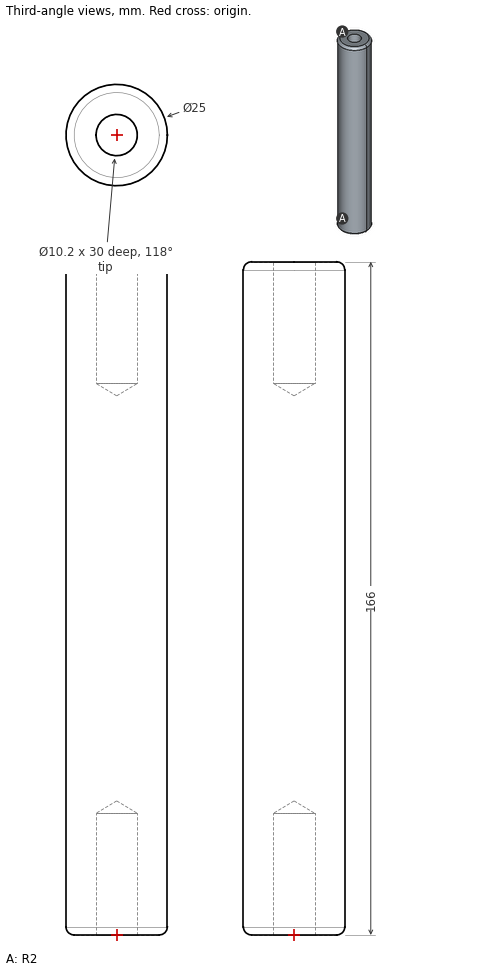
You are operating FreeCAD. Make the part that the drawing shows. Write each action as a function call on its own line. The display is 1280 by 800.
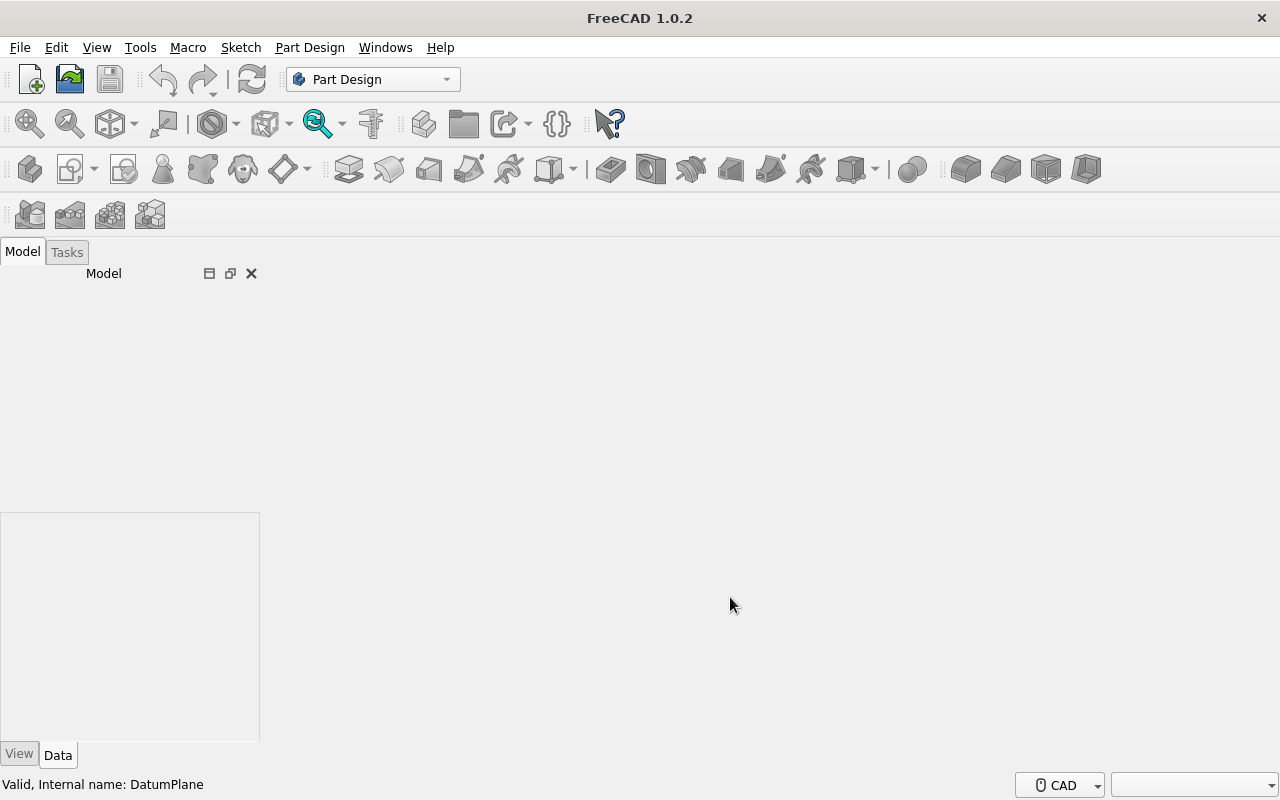
click(30, 80)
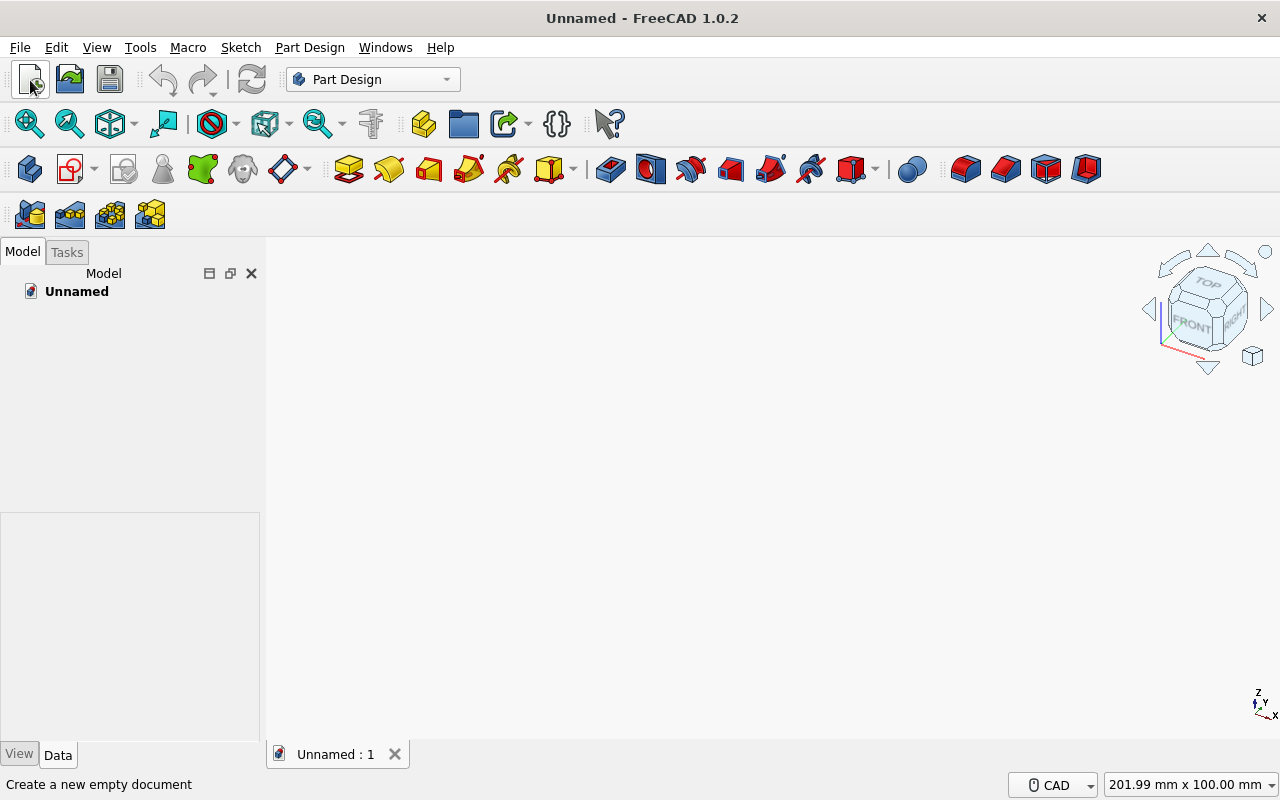
click(70, 170)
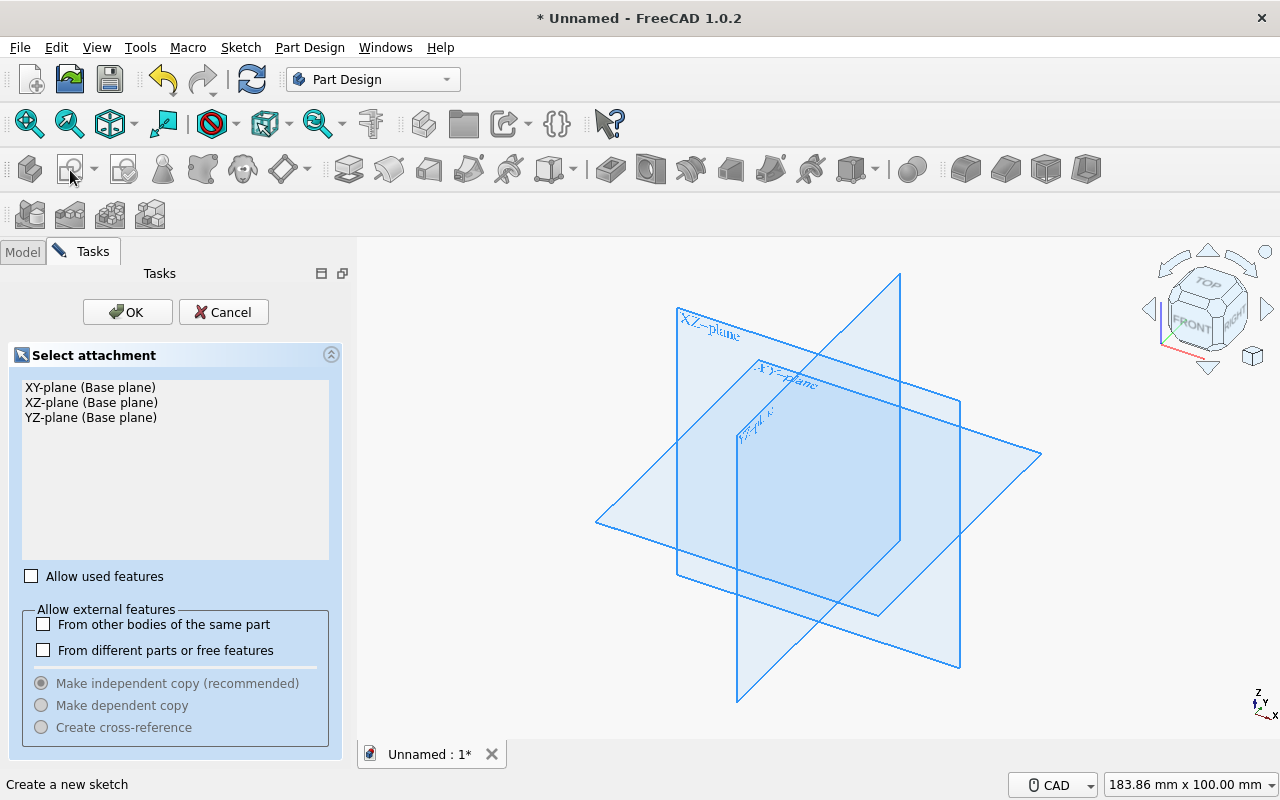
click(82, 388)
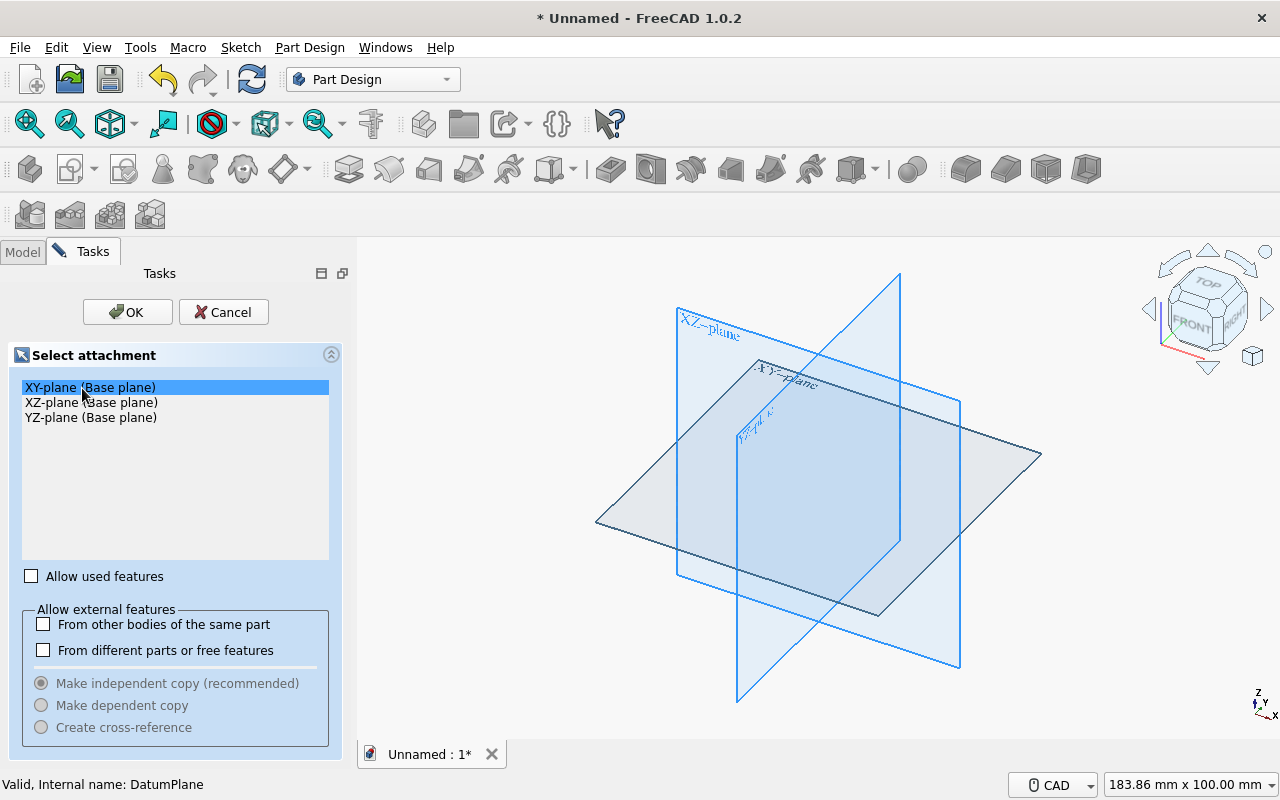
click(128, 312)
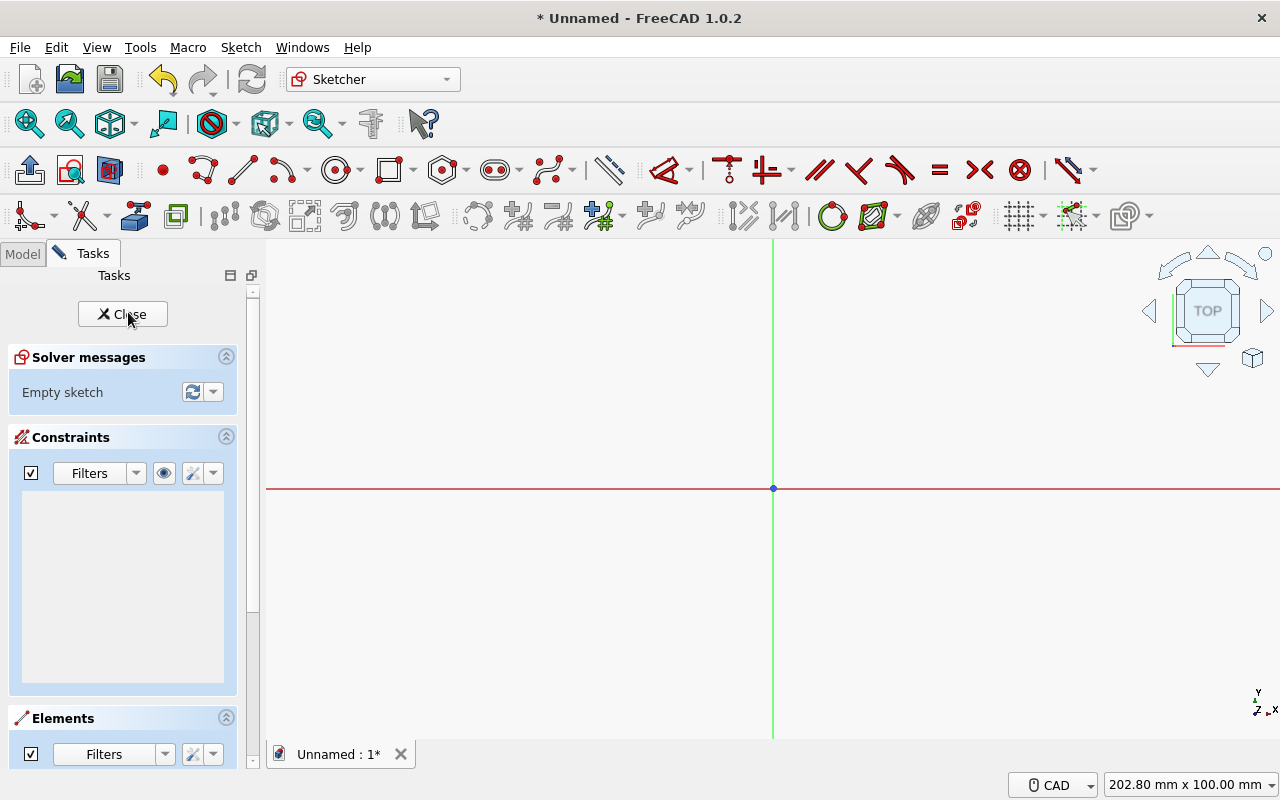
scroll(813, 489, up, 5)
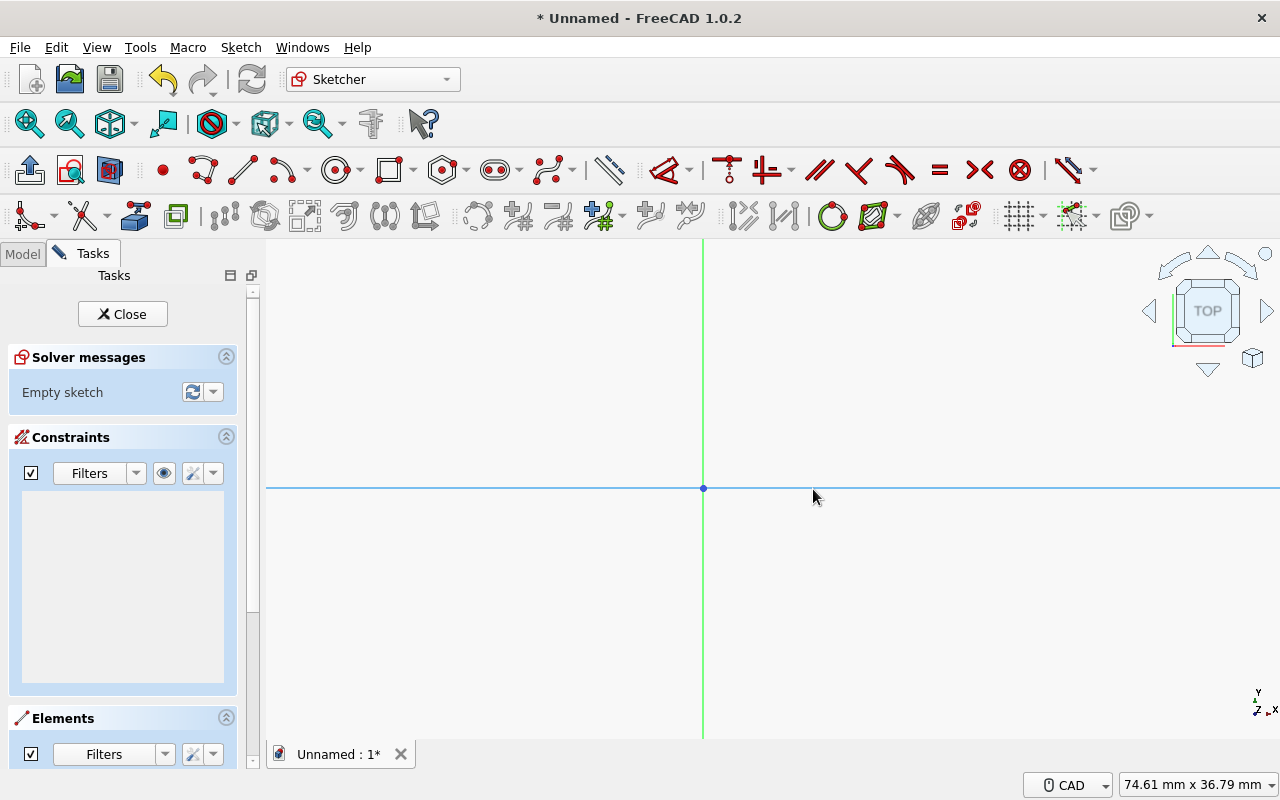
click(336, 170)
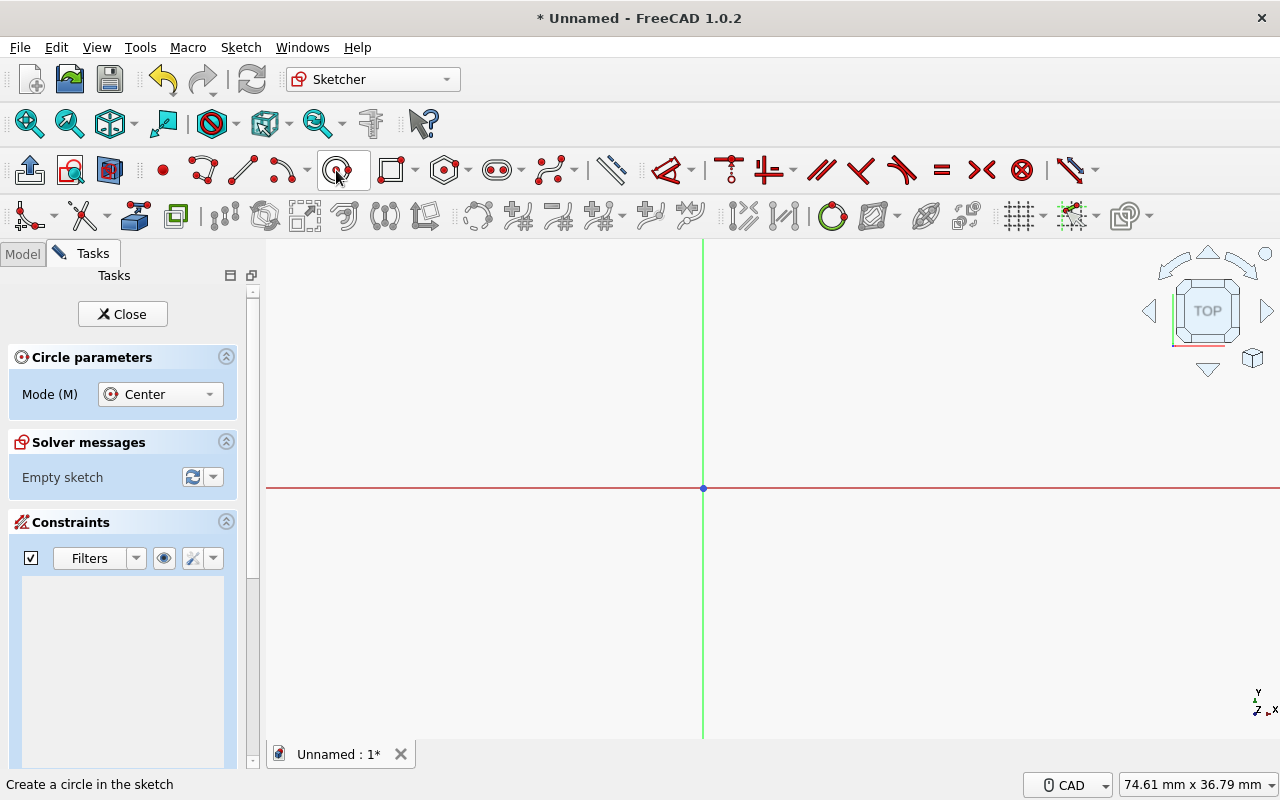
click(703, 488)
click(823, 368)
key(Escape)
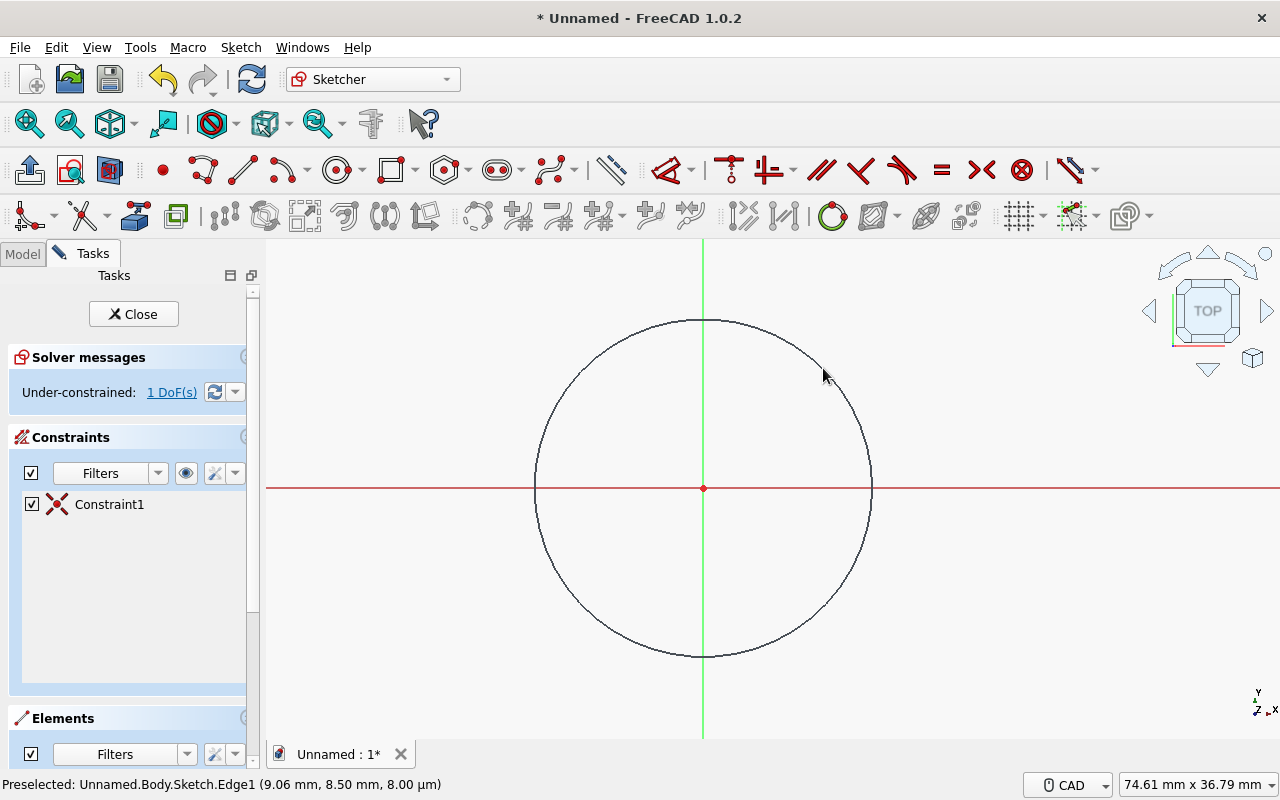
click(666, 170)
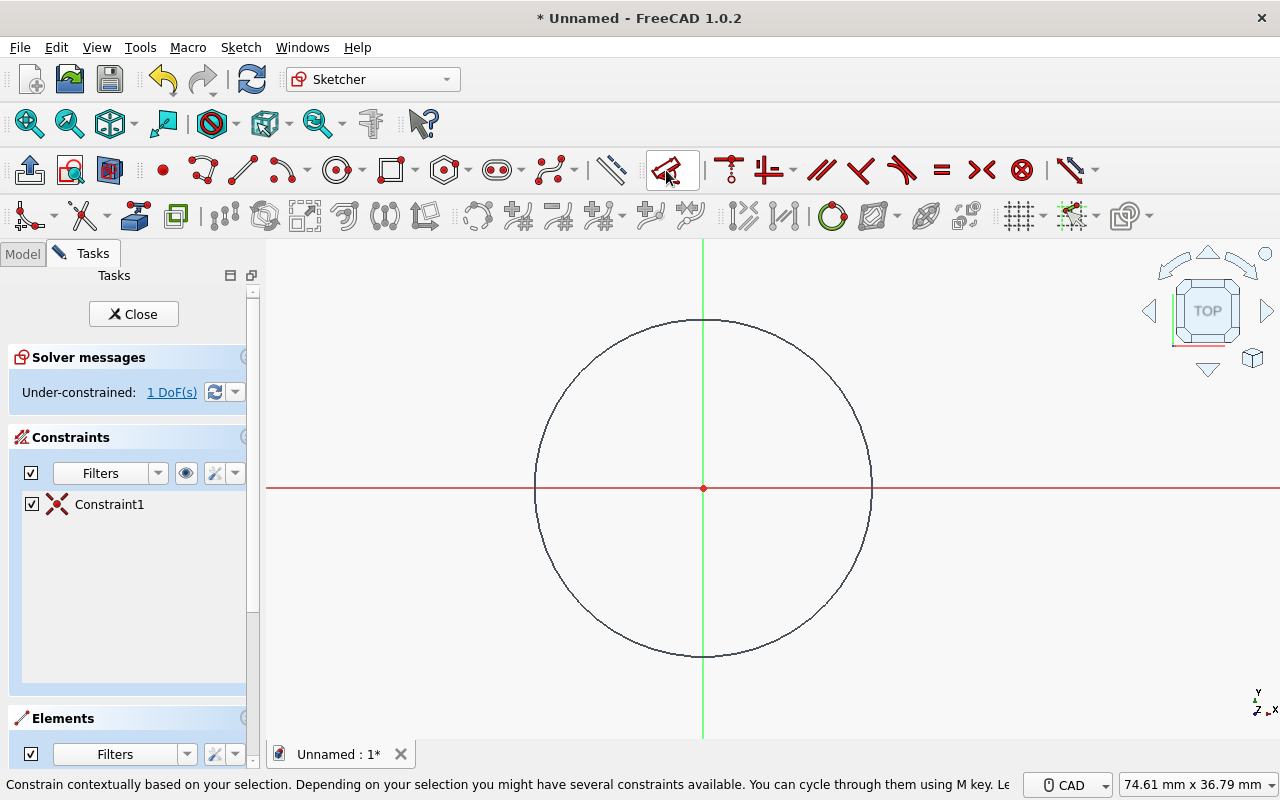
click(822, 368)
click(844, 345)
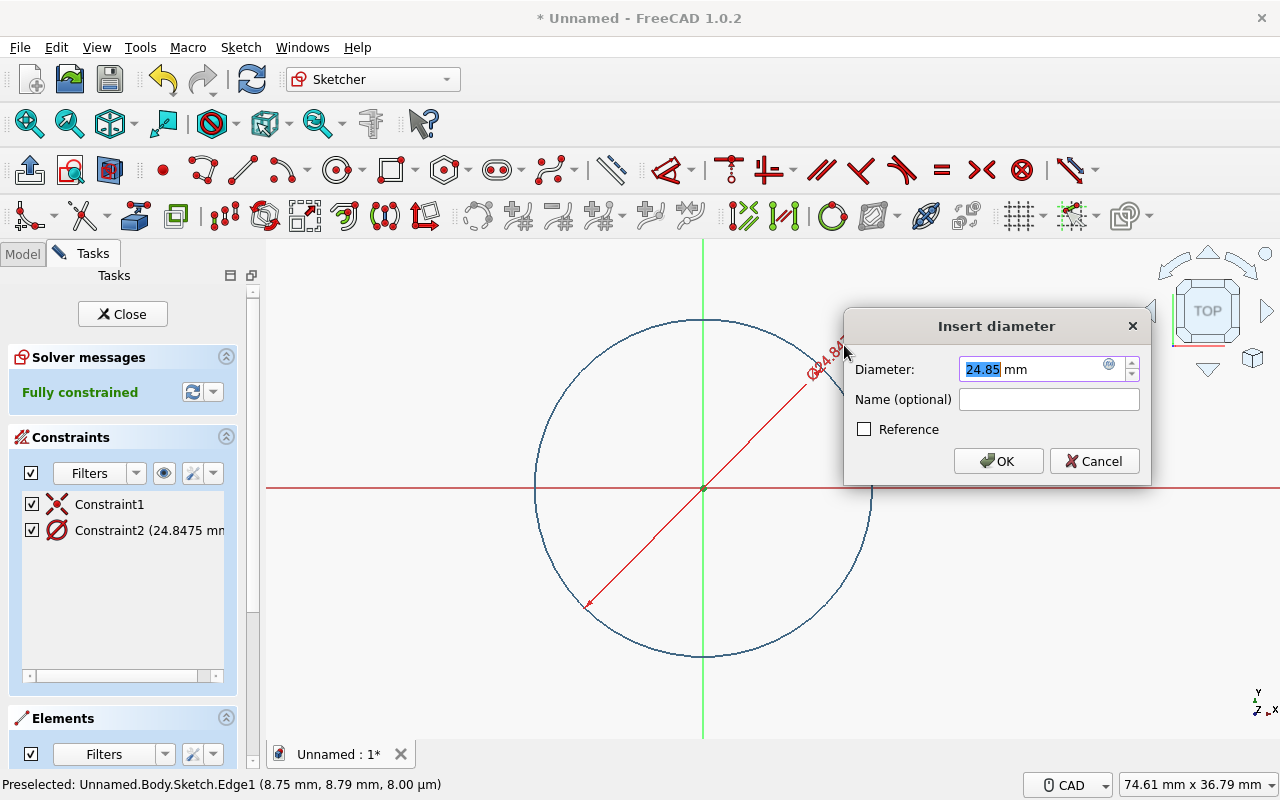
text(25)
key(Return)
key(Escape)